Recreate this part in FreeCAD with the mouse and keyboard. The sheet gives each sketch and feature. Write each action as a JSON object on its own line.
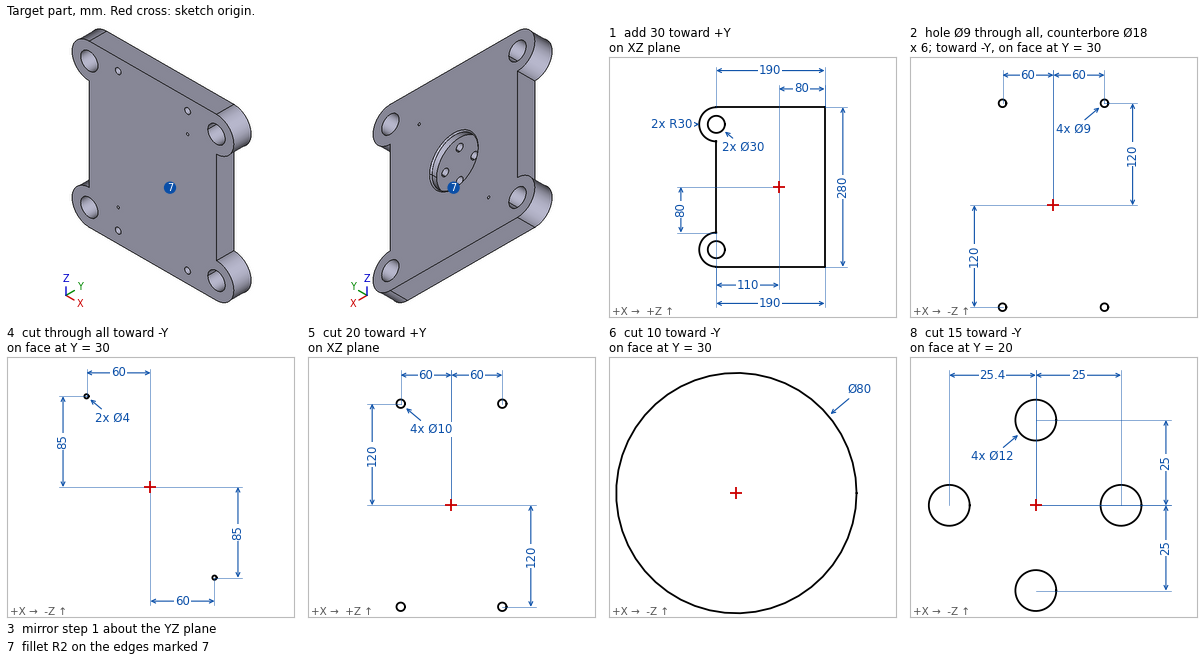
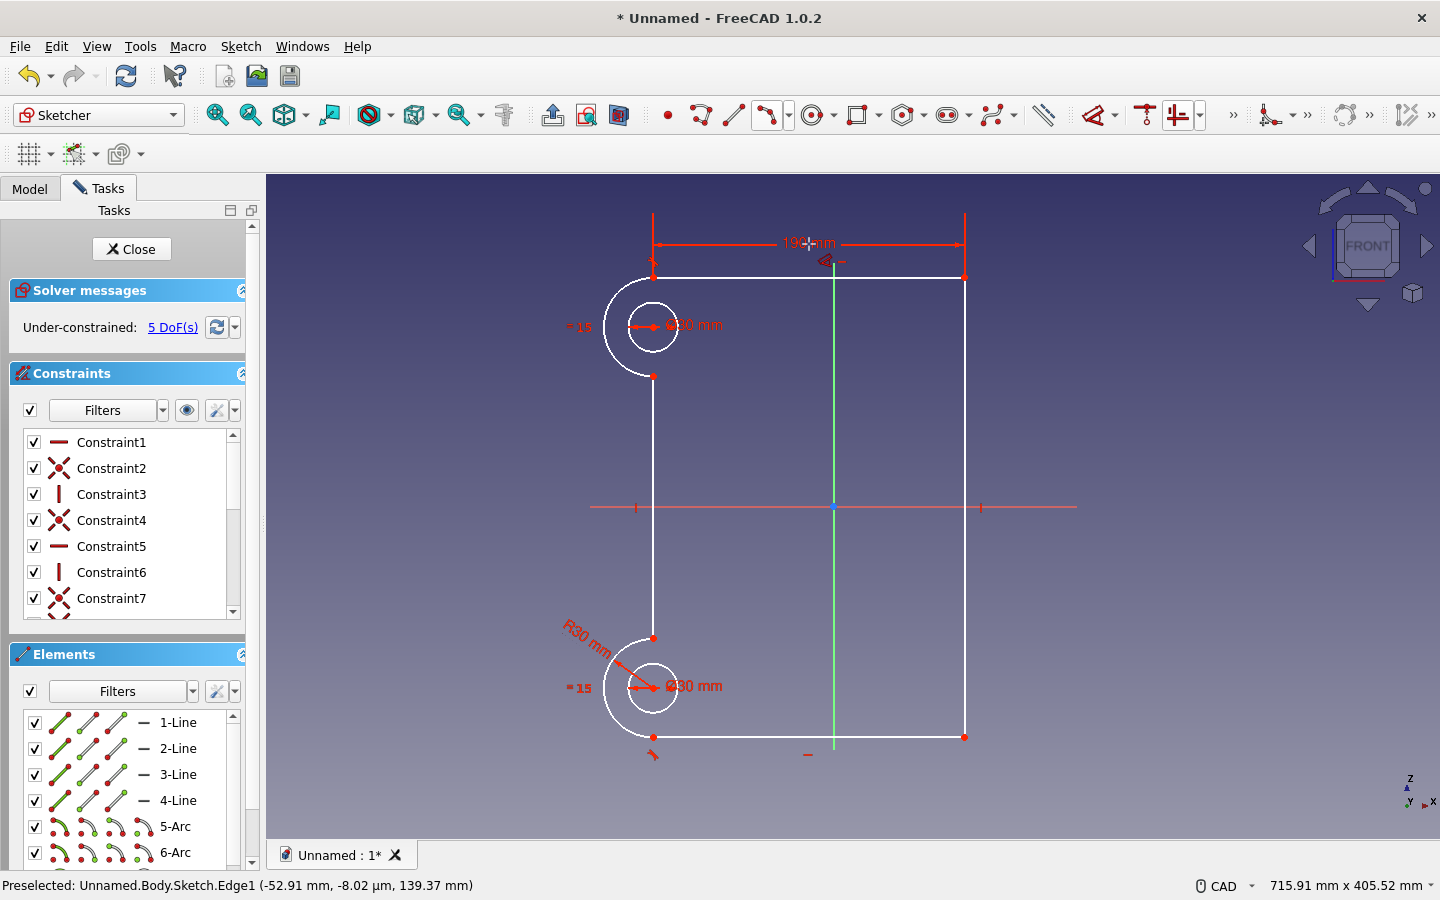
{"action": "left_click", "coordinate": [965, 416]}
{"action": "left_click", "coordinate": [999, 402]}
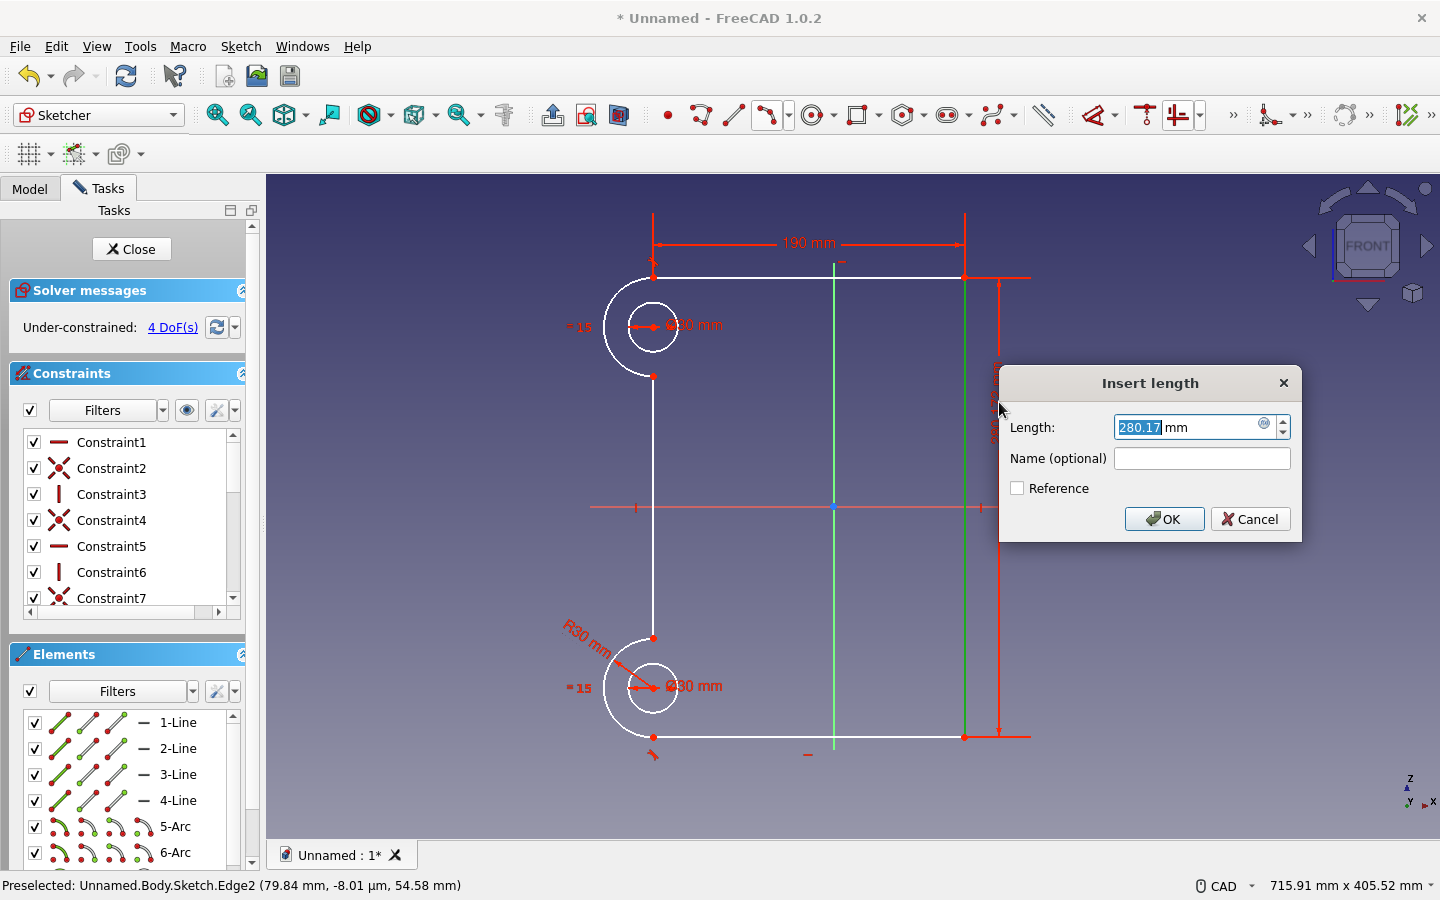
{"action": "type", "text": "280"}
{"action": "key", "text": "Return"}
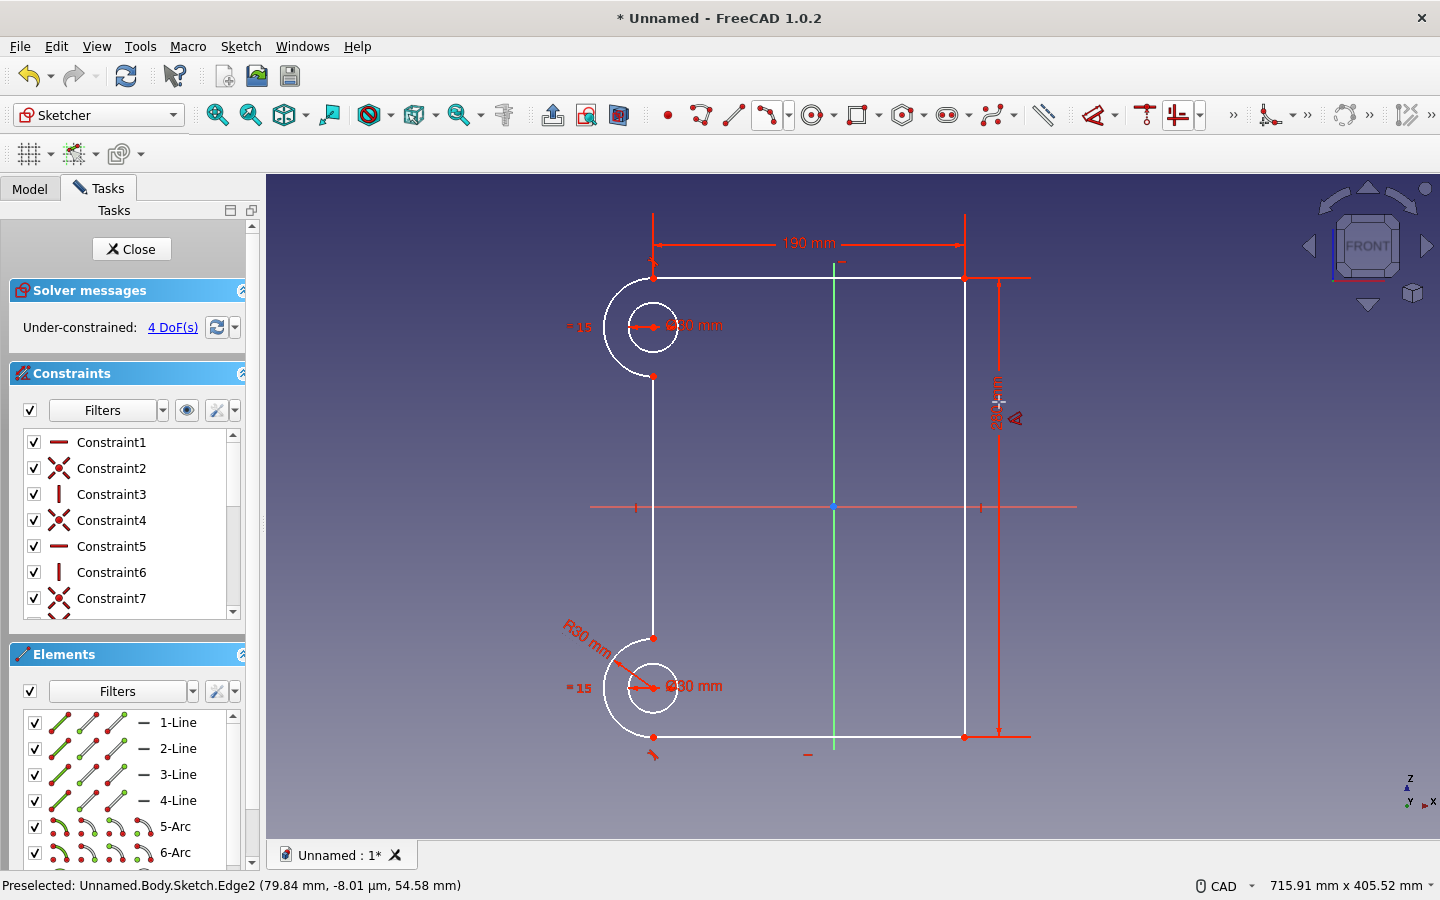
{"action": "left_click", "coordinate": [871, 737]}
{"action": "left_click", "coordinate": [809, 771]}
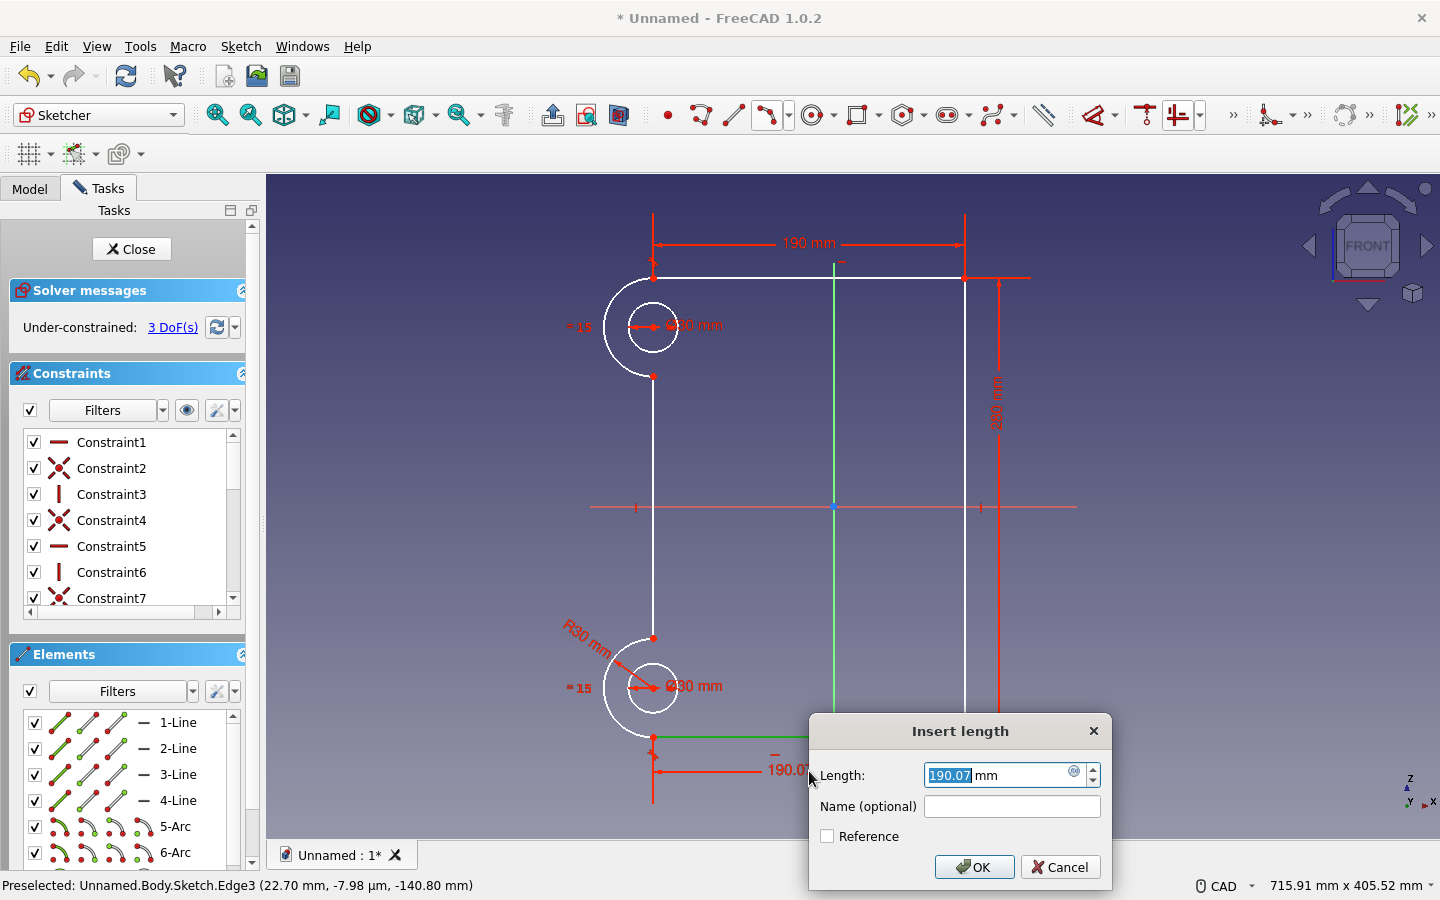
{"action": "type", "text": "190"}
{"action": "key", "text": "Return"}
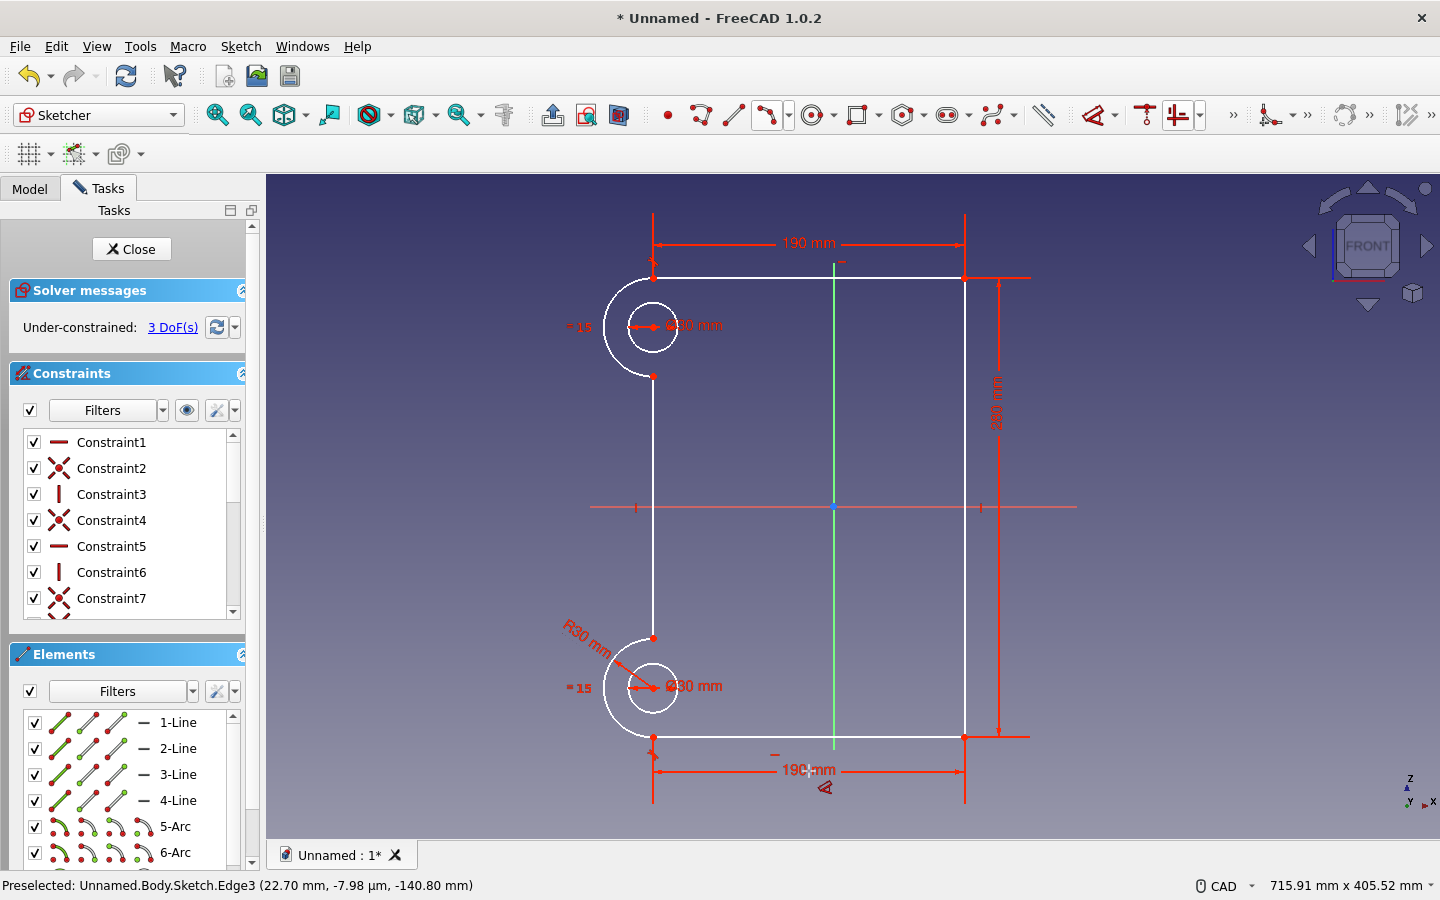
{"action": "left_click", "coordinate": [965, 278]}
{"action": "left_click", "coordinate": [899, 244]}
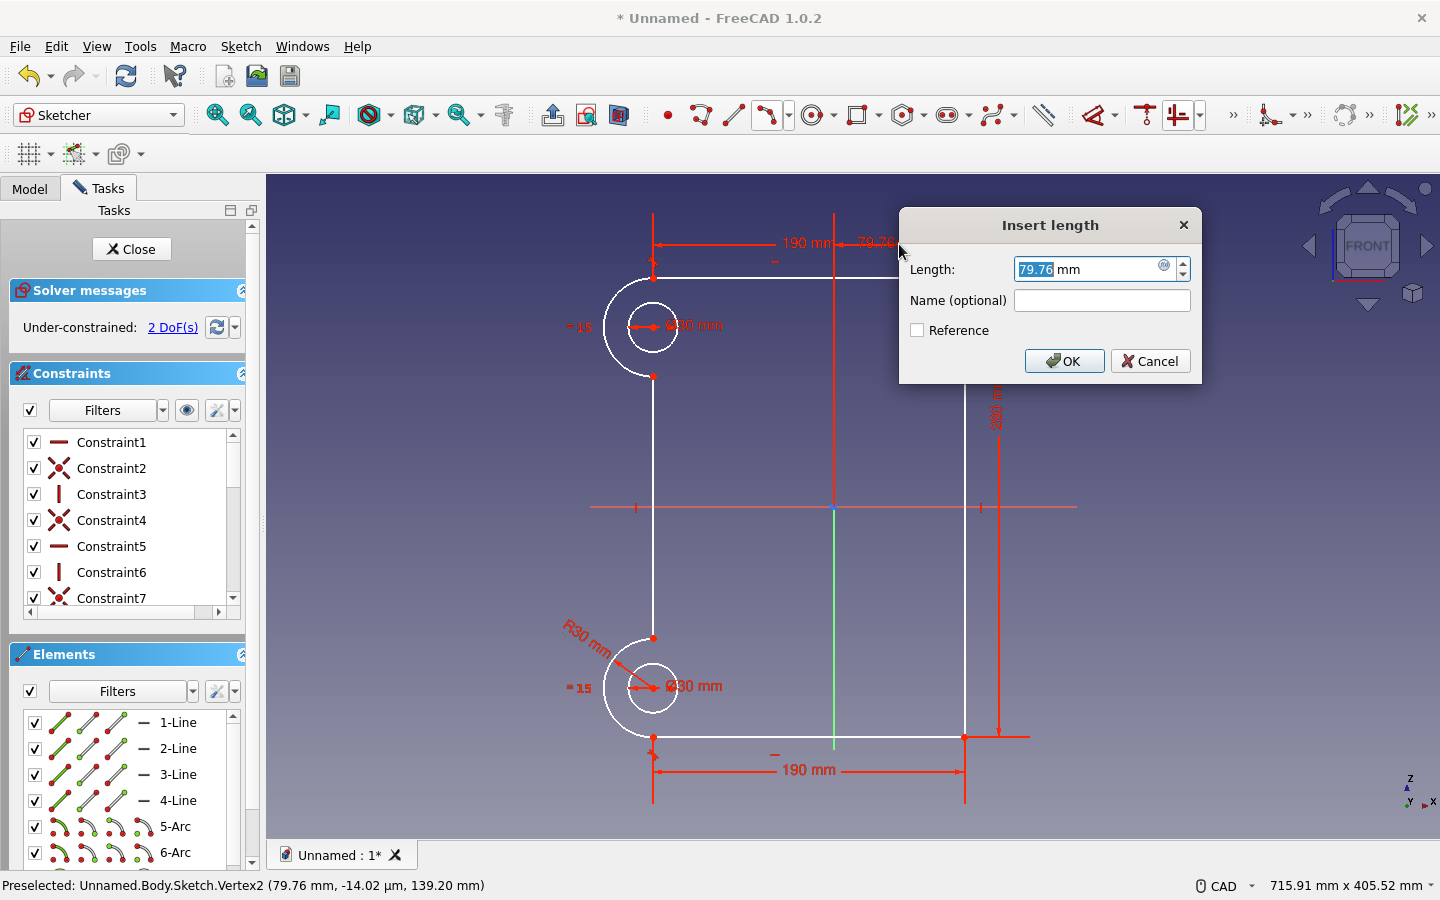
{"action": "type", "text": "80"}
{"action": "key", "text": "Return"}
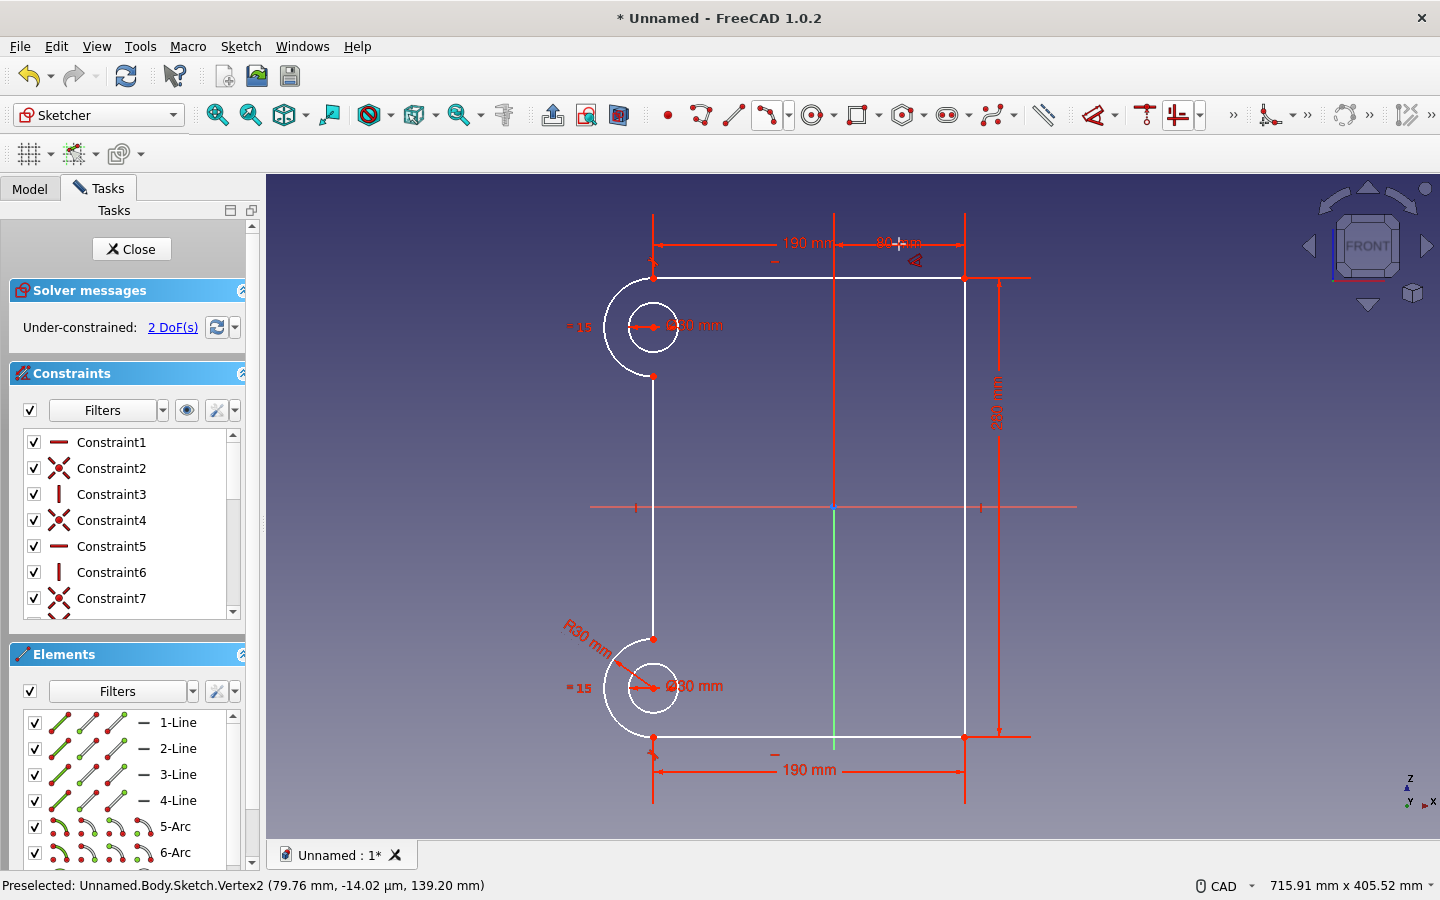
{"action": "left_click", "coordinate": [653, 639]}
{"action": "left_click", "coordinate": [619, 573]}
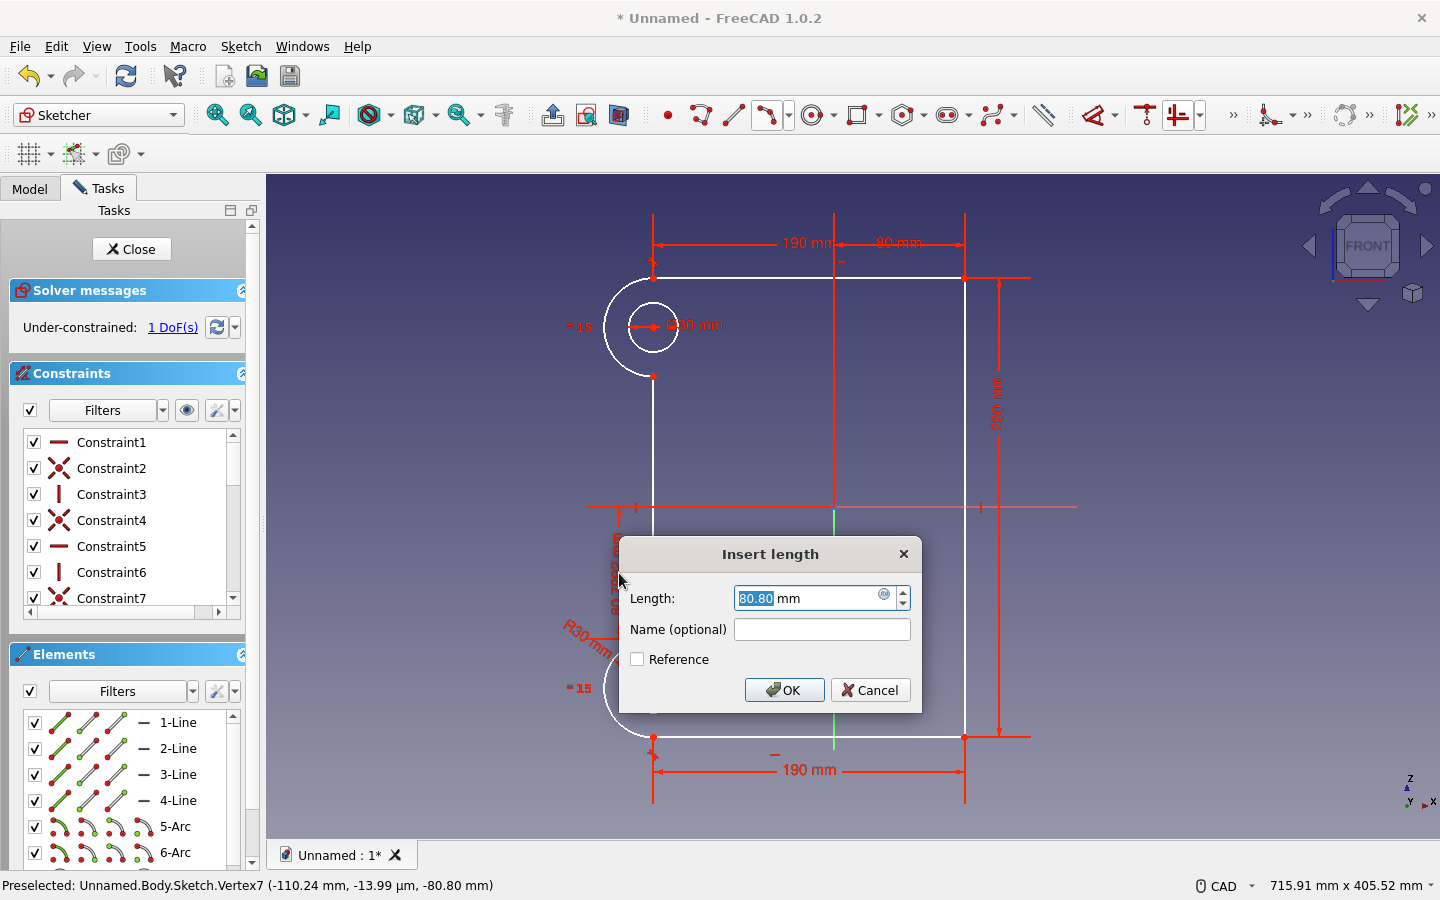
{"action": "type", "text": "80"}
{"action": "key", "text": "Return"}